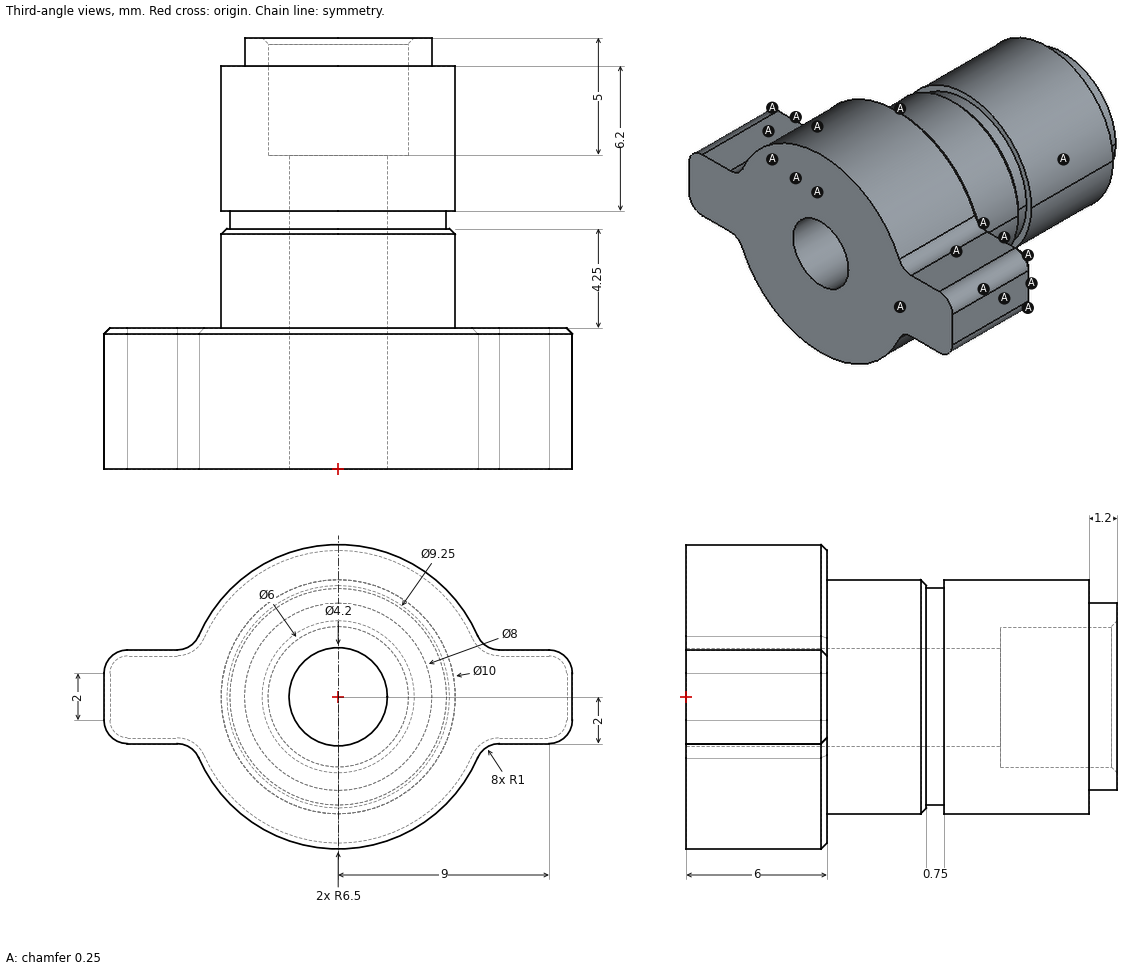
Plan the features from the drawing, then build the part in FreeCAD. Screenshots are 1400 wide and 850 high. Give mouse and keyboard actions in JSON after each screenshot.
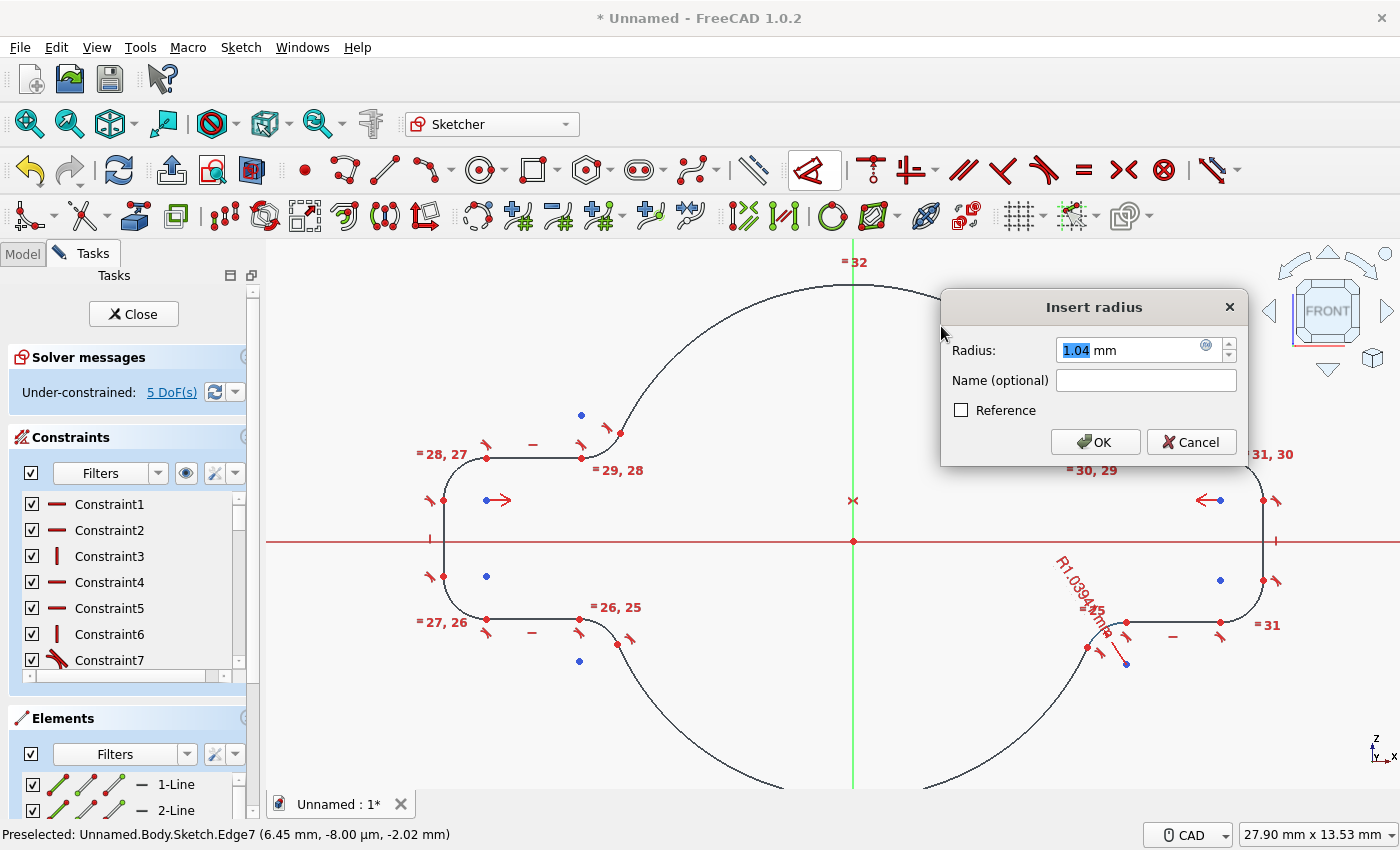
{"action": "type", "text": "1"}
{"action": "key", "text": "Return"}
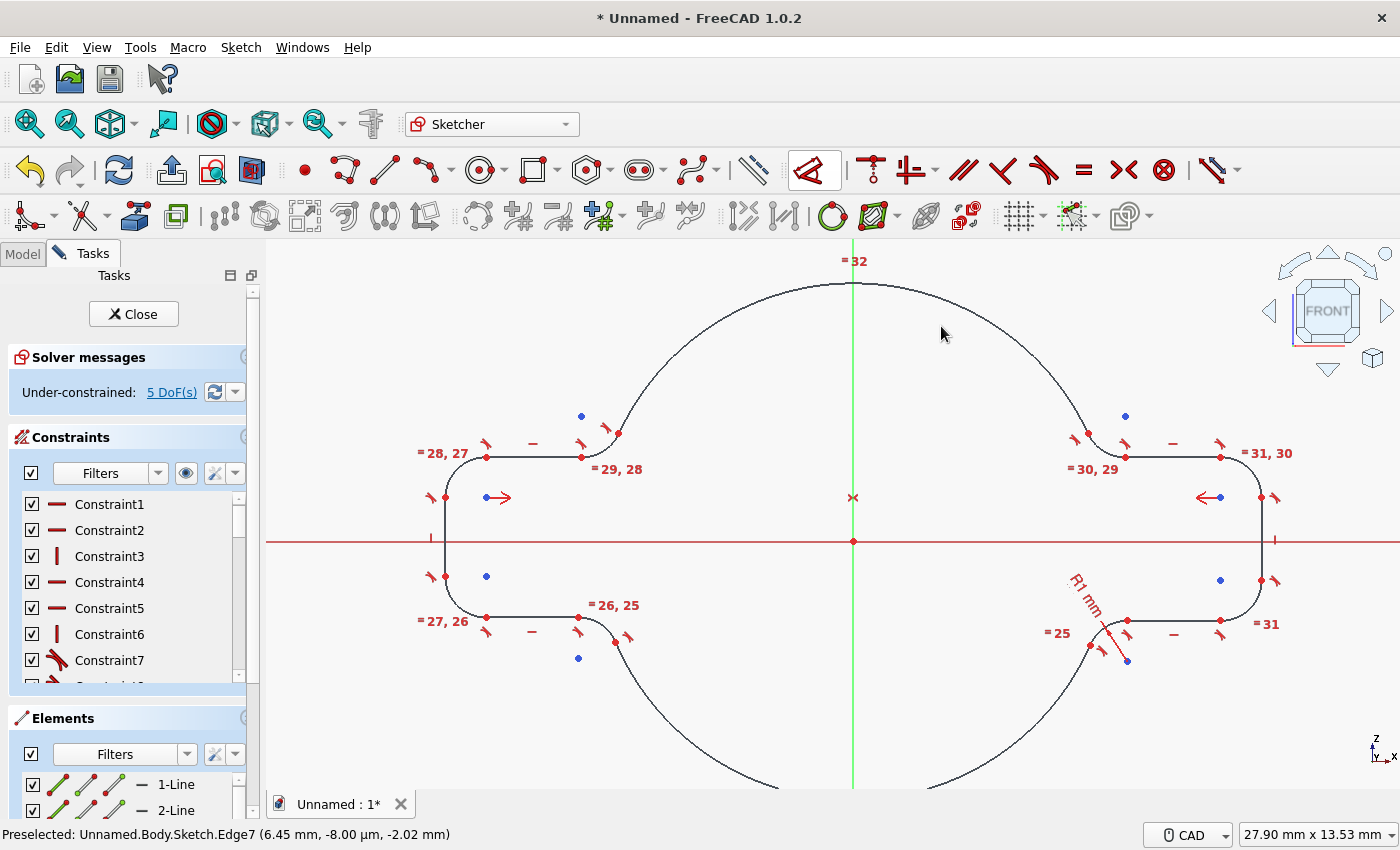
{"action": "left_click", "coordinate": [686, 738]}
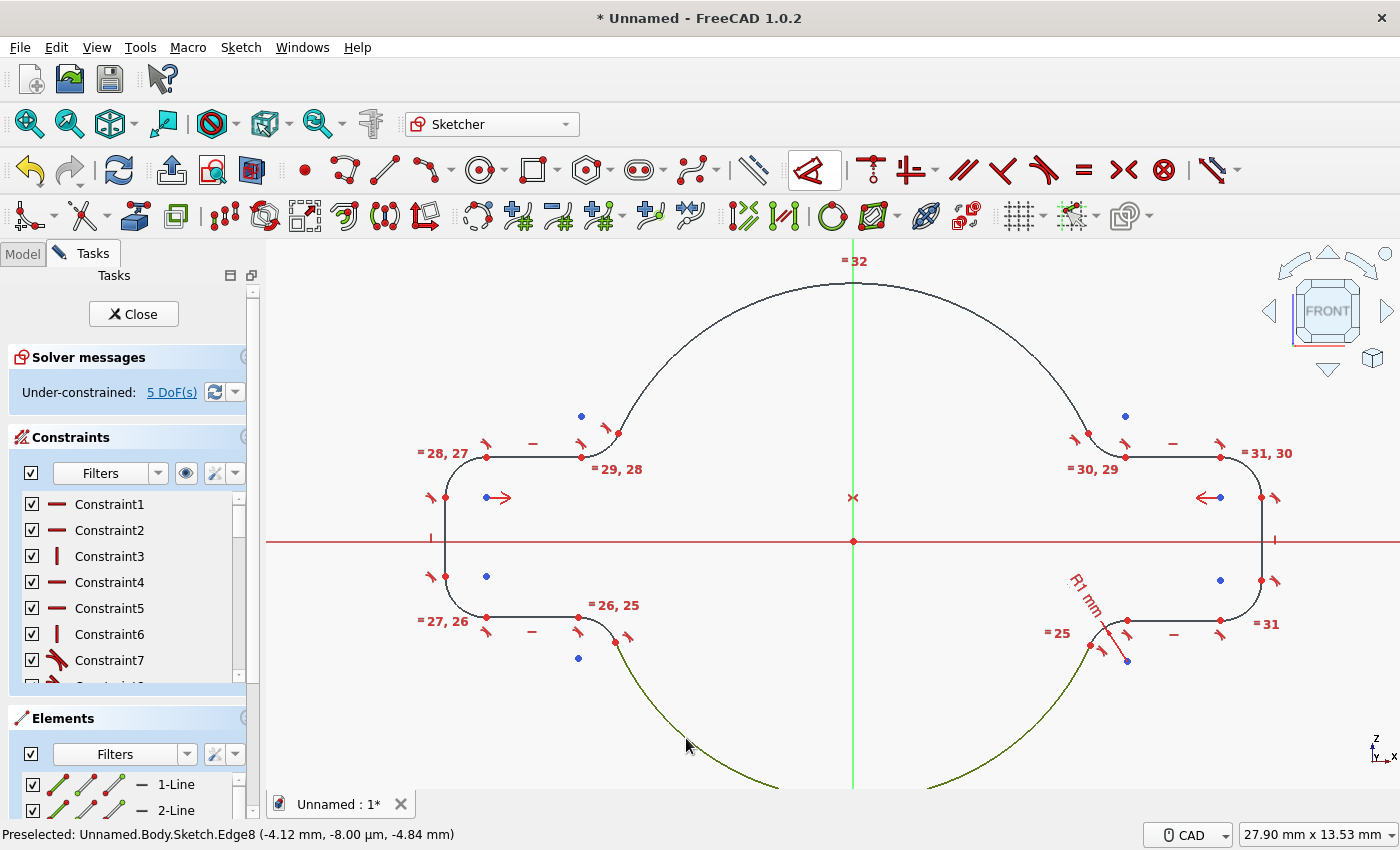
{"action": "key", "text": "k r"}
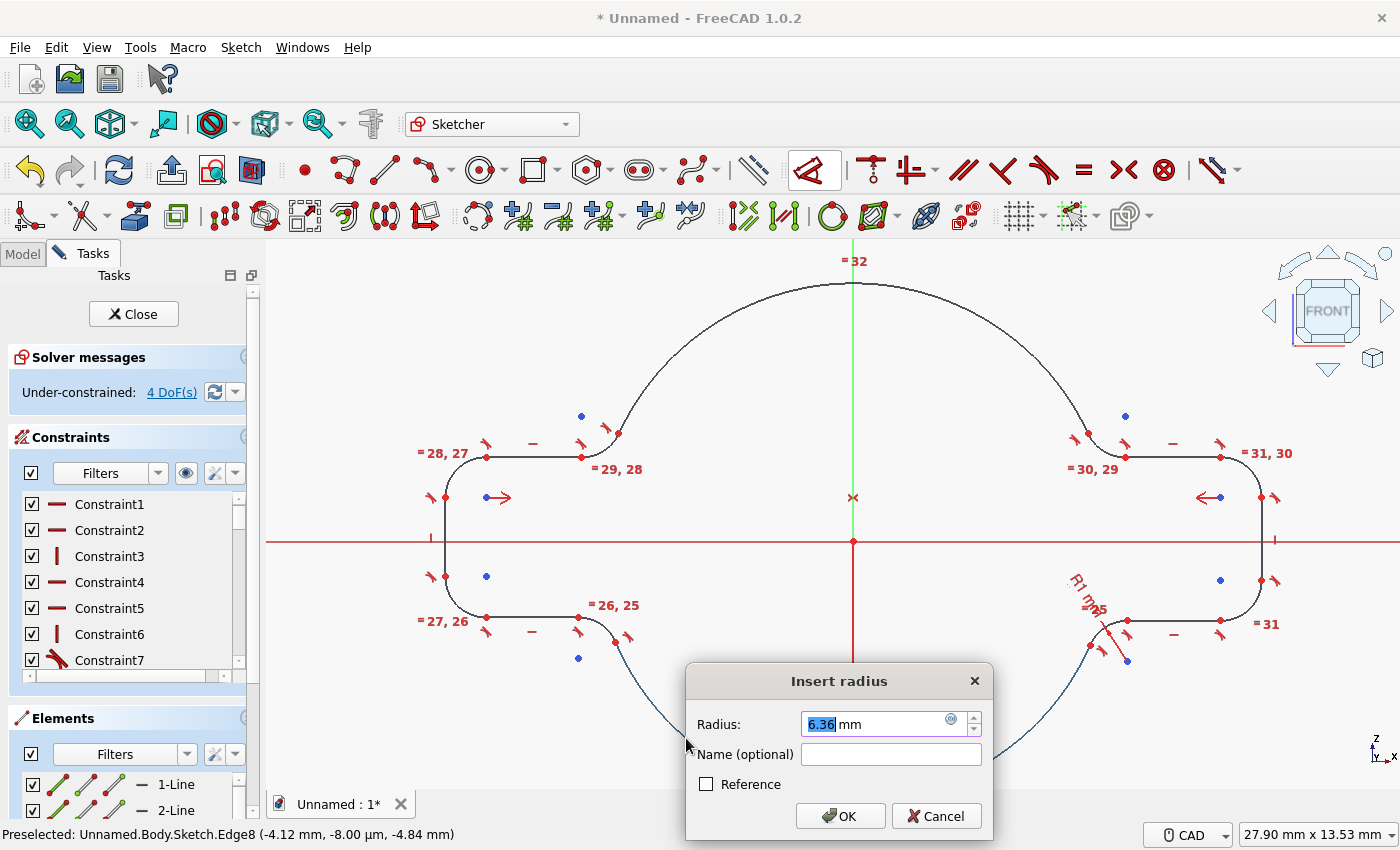
{"action": "type", "text": "6.5"}
{"action": "key", "text": "Return"}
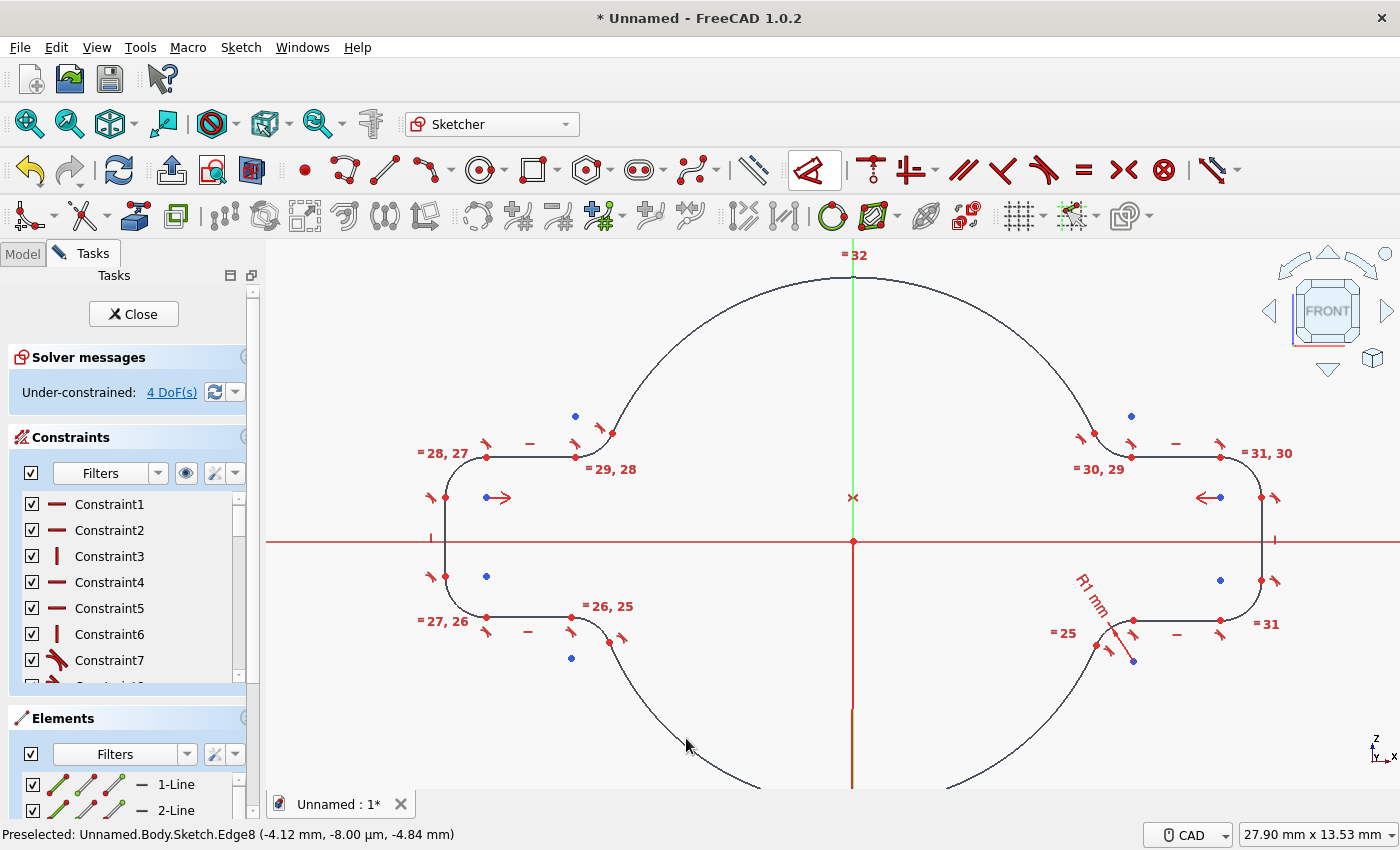
{"action": "left_click", "coordinate": [445, 553]}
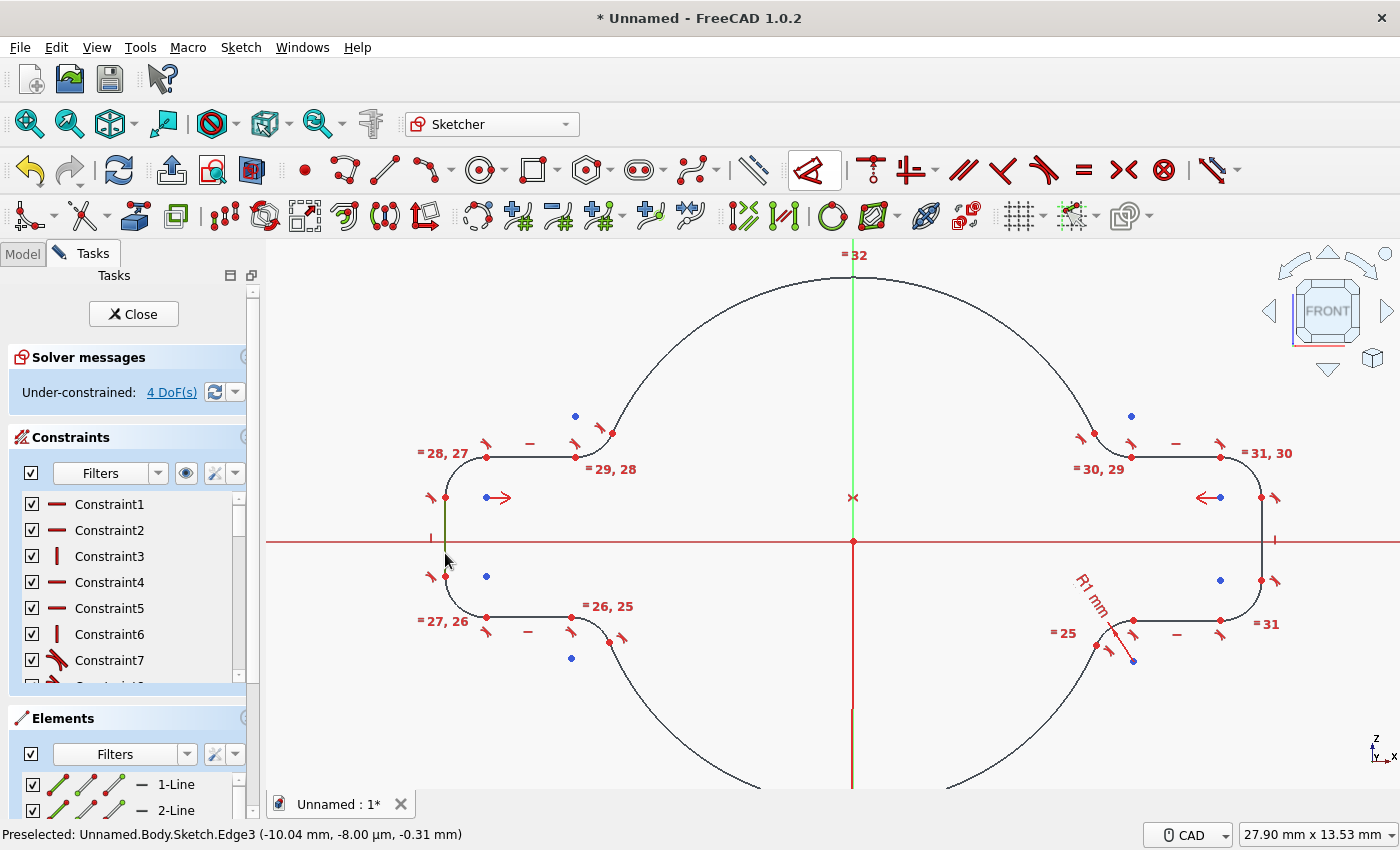
{"action": "left_click", "coordinate": [836, 170]}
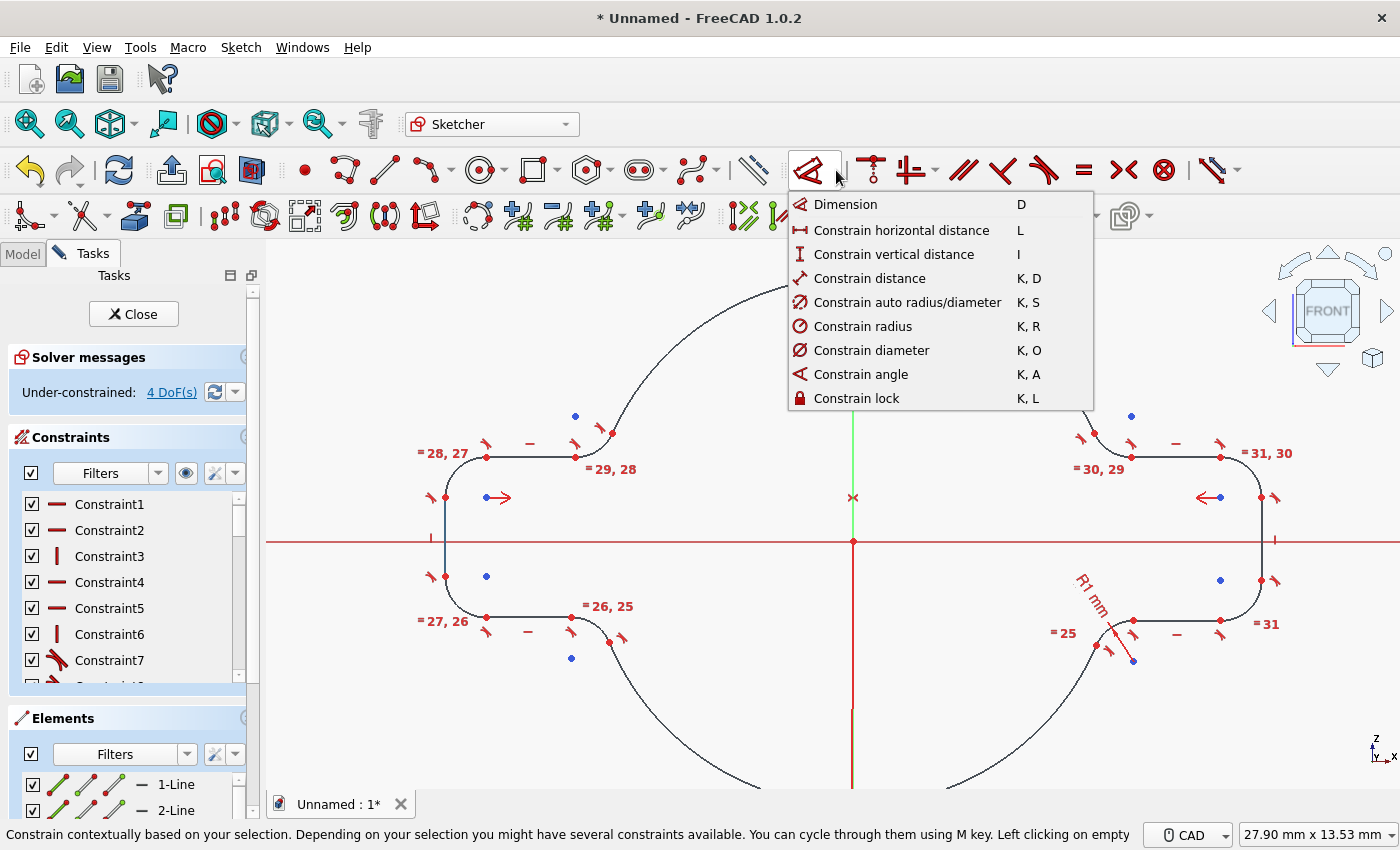
{"action": "left_click", "coordinate": [941, 254]}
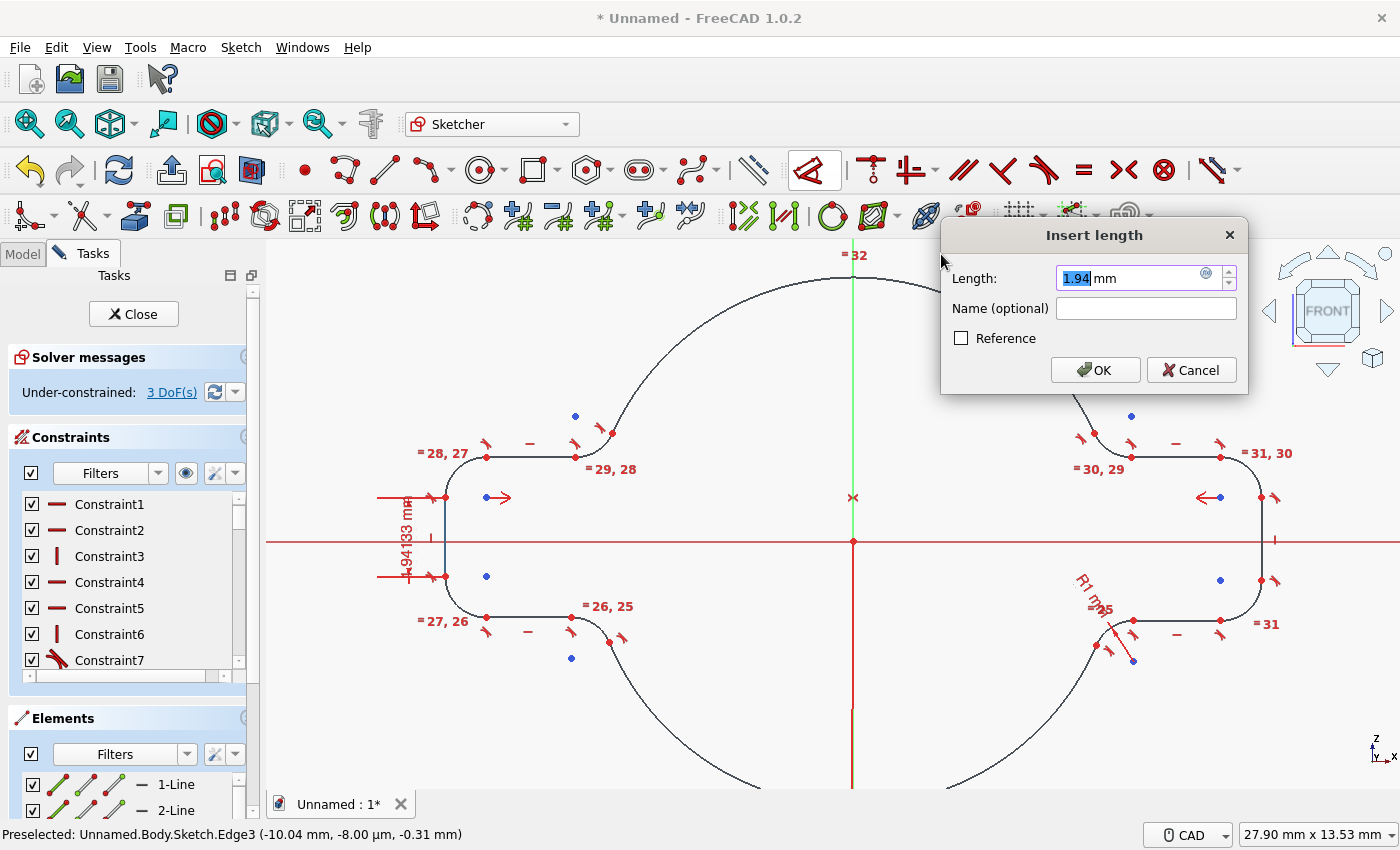
{"action": "type", "text": "2"}
{"action": "key", "text": "Return"}